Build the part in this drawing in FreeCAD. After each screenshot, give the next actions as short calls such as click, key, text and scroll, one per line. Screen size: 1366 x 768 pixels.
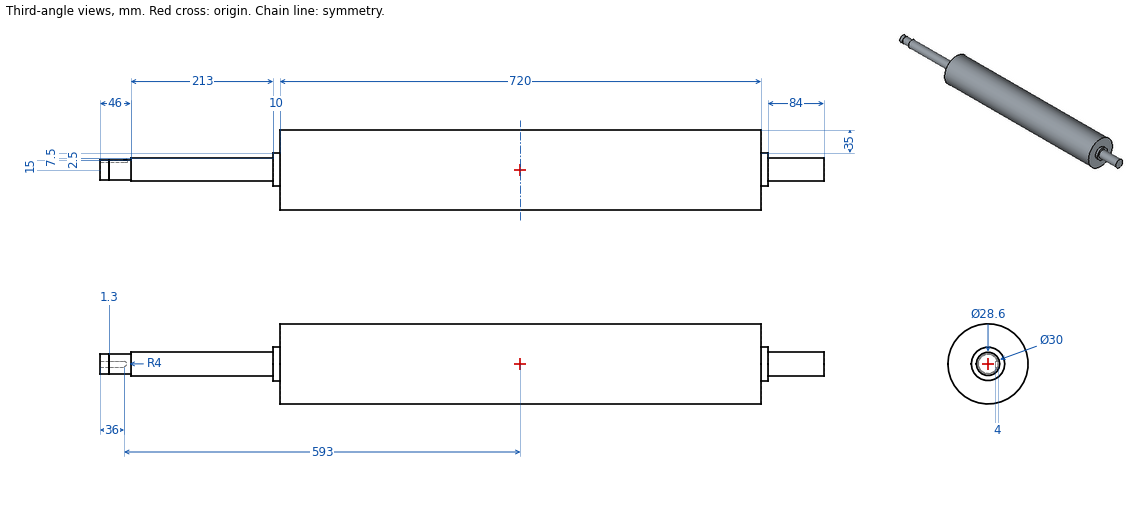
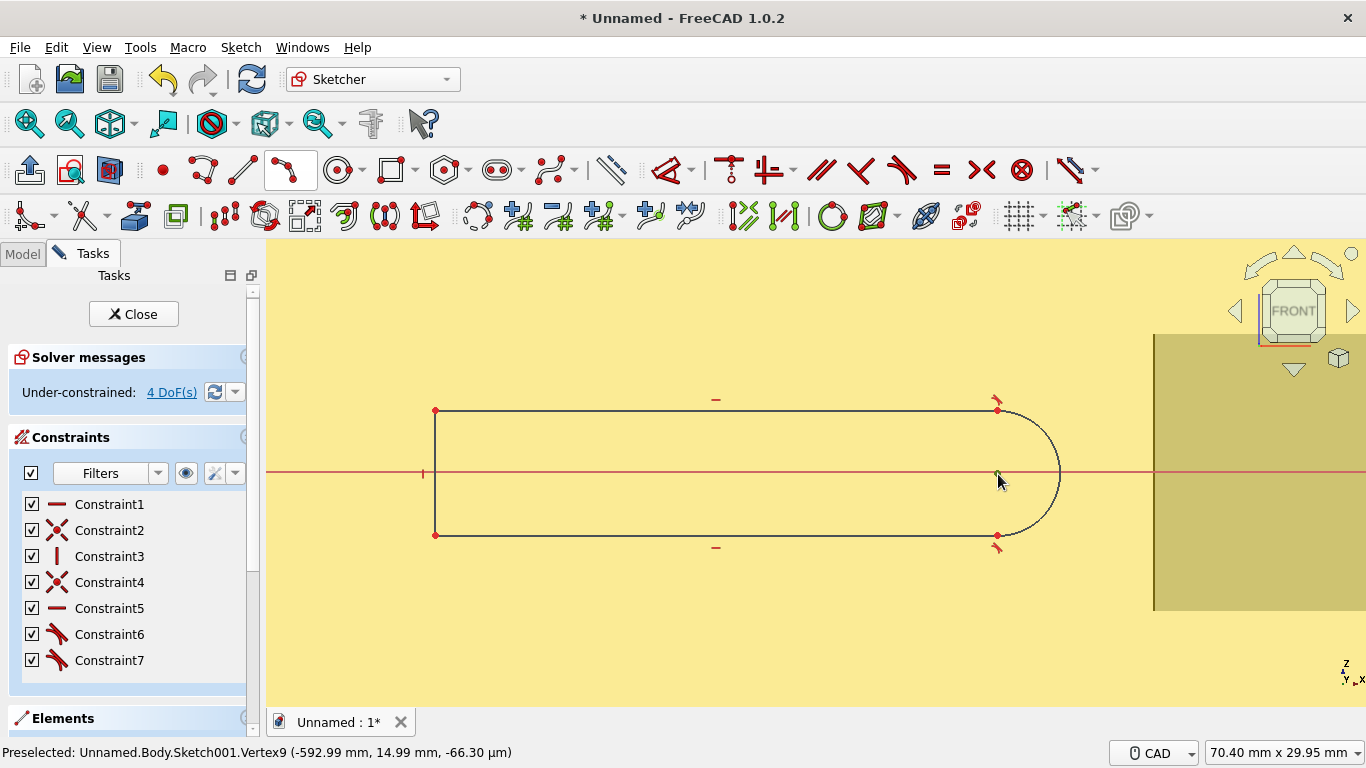
click(359, 472)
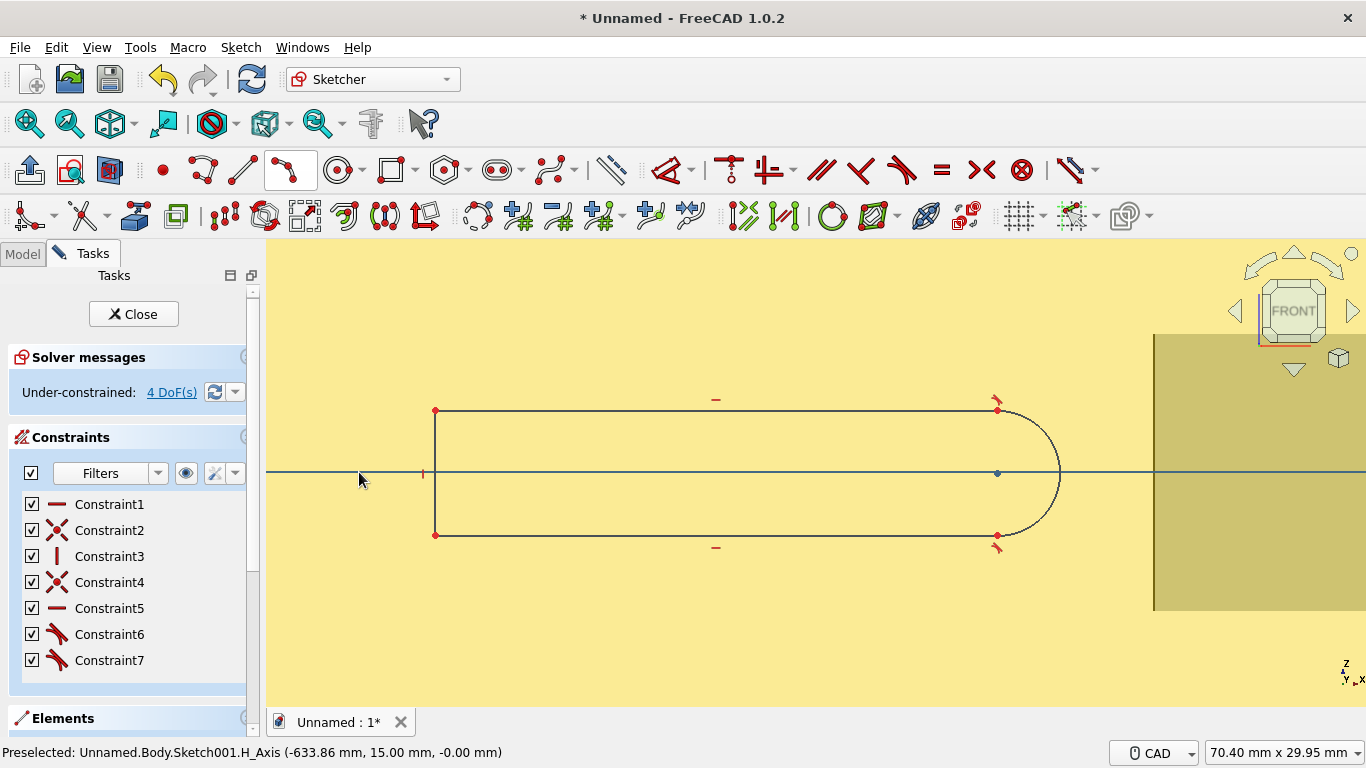
click(730, 170)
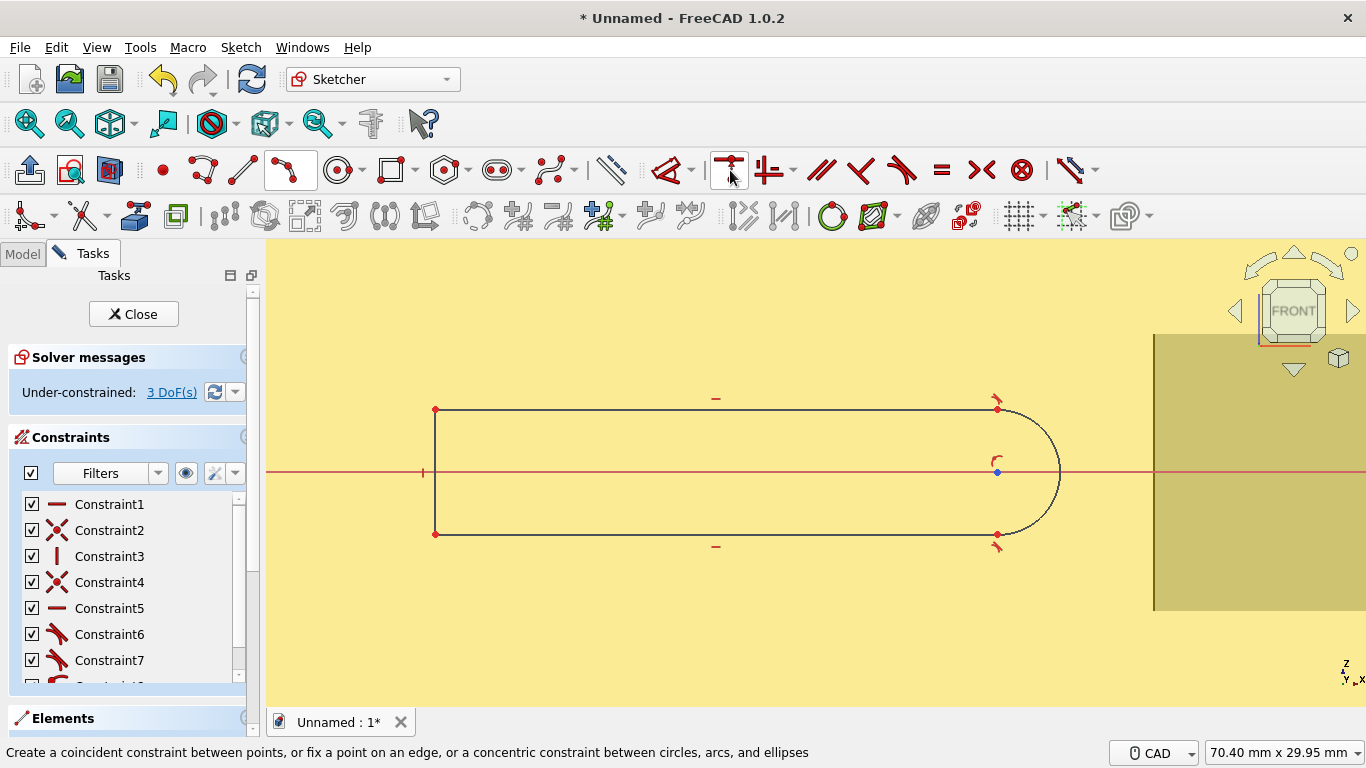
click(666, 170)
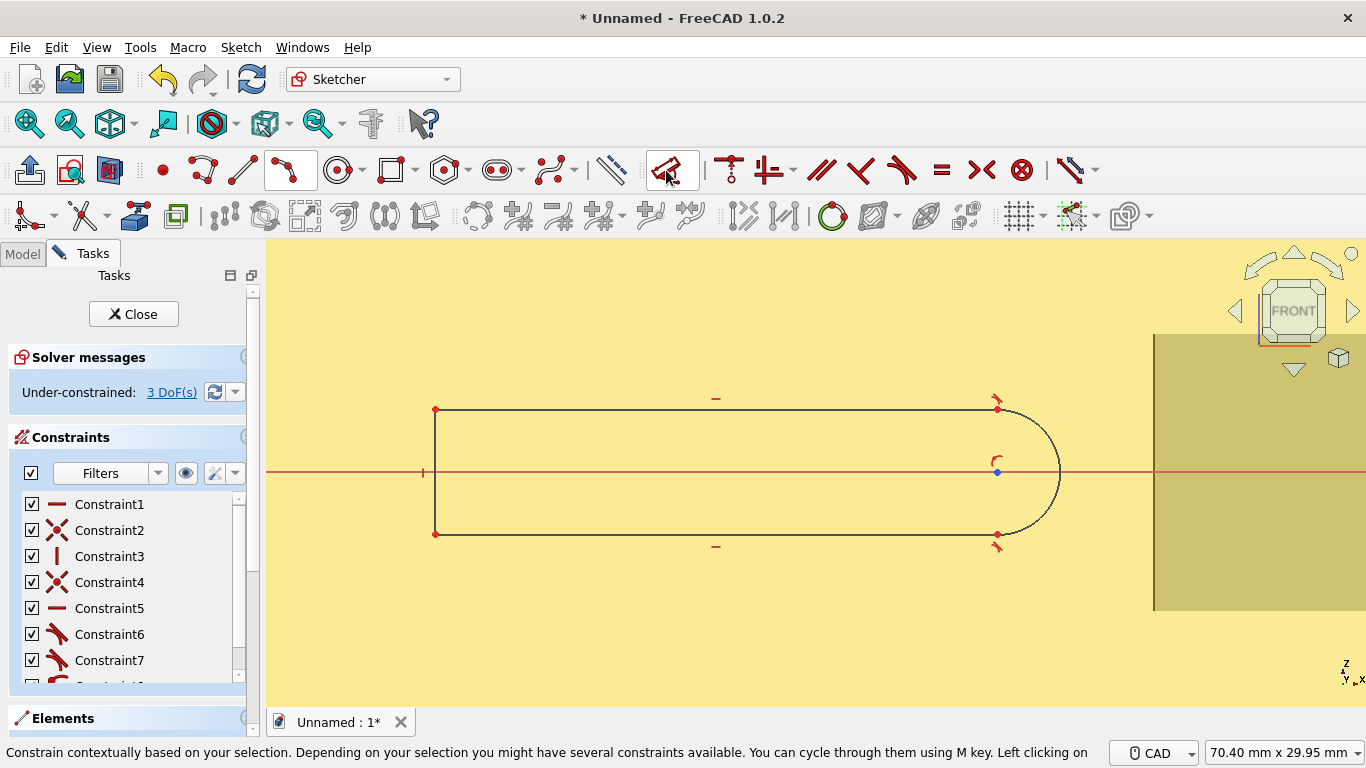
click(1048, 509)
click(1074, 528)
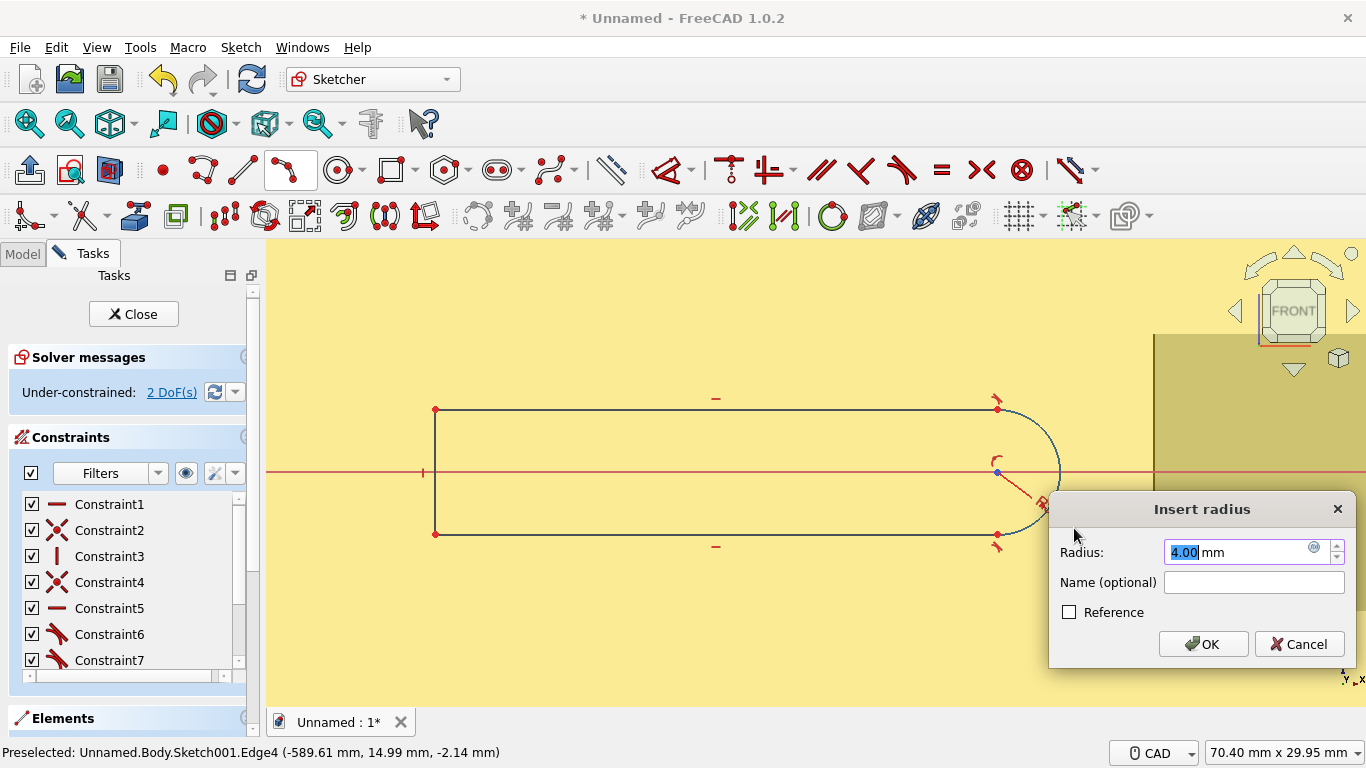
text(4)
key(Return)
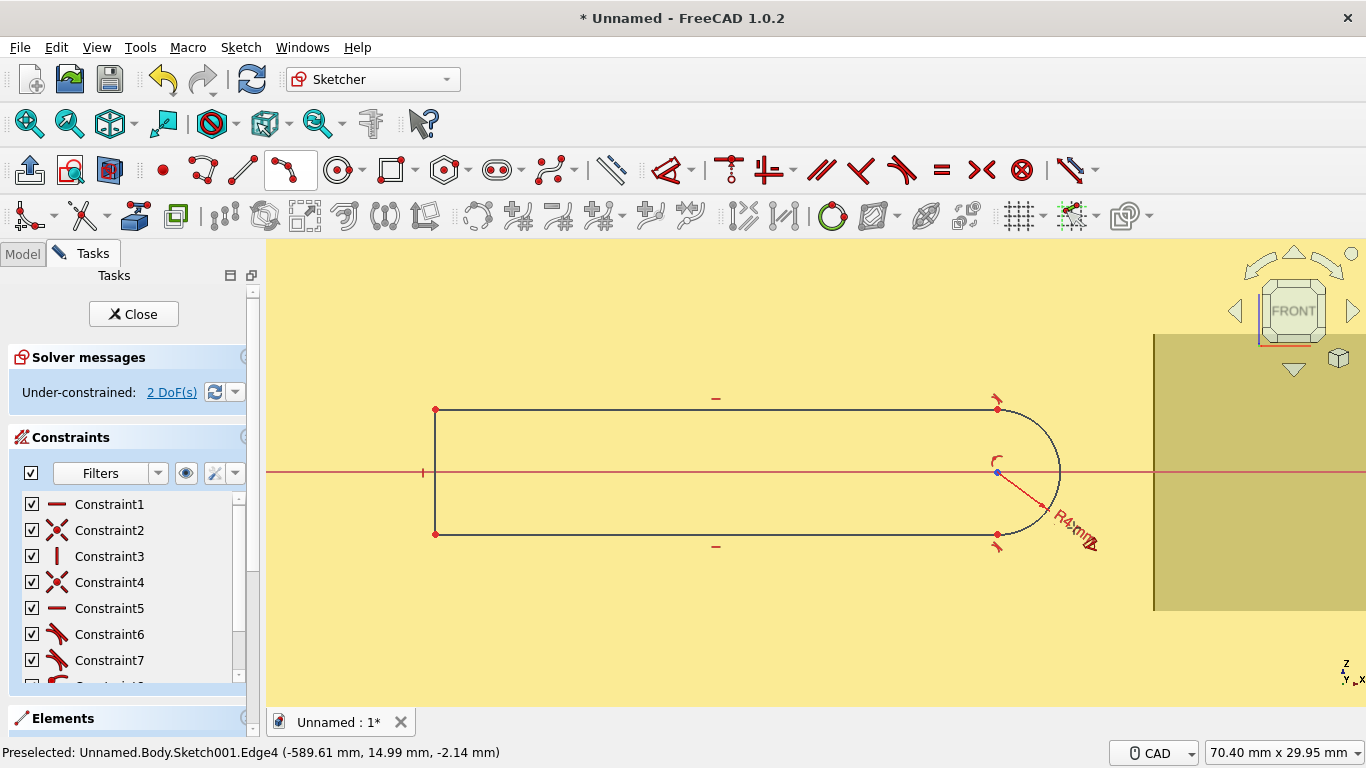
click(829, 535)
click(716, 569)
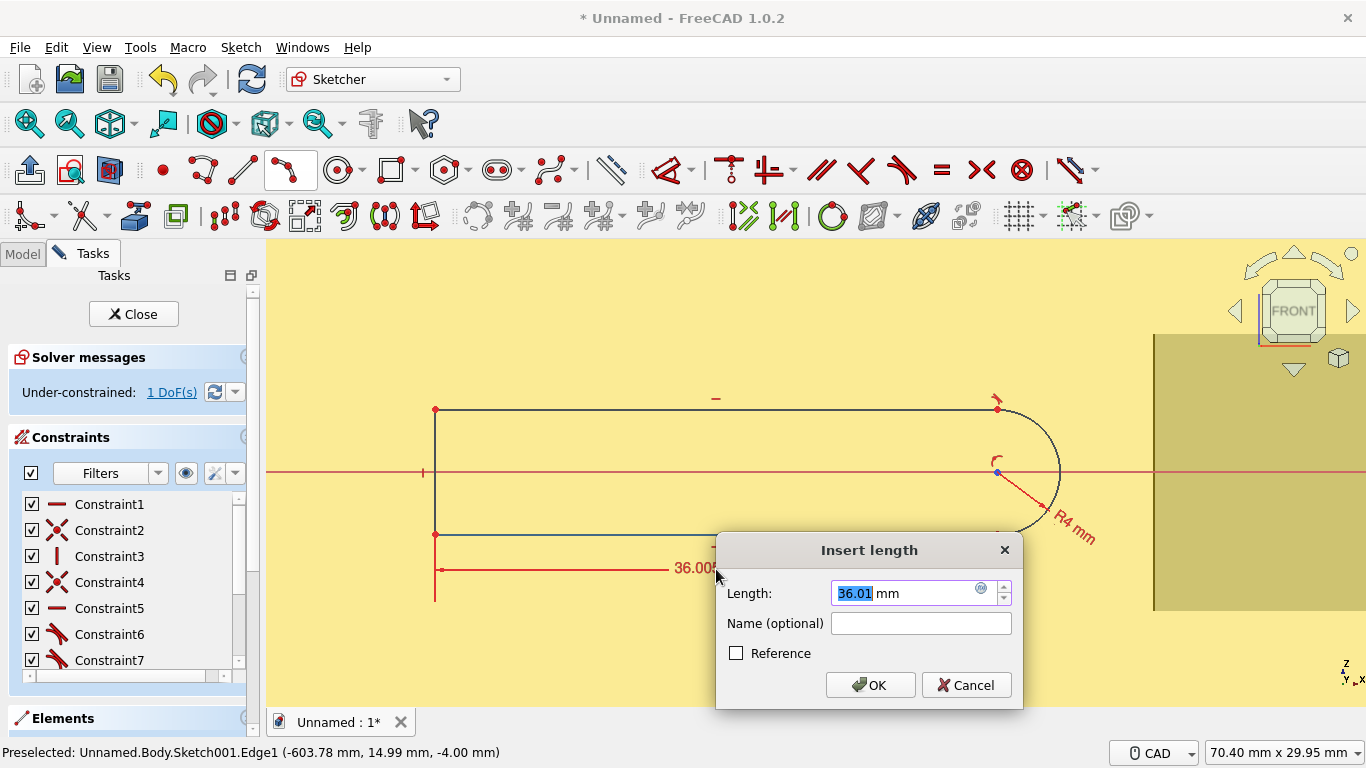
text(36)
key(Return)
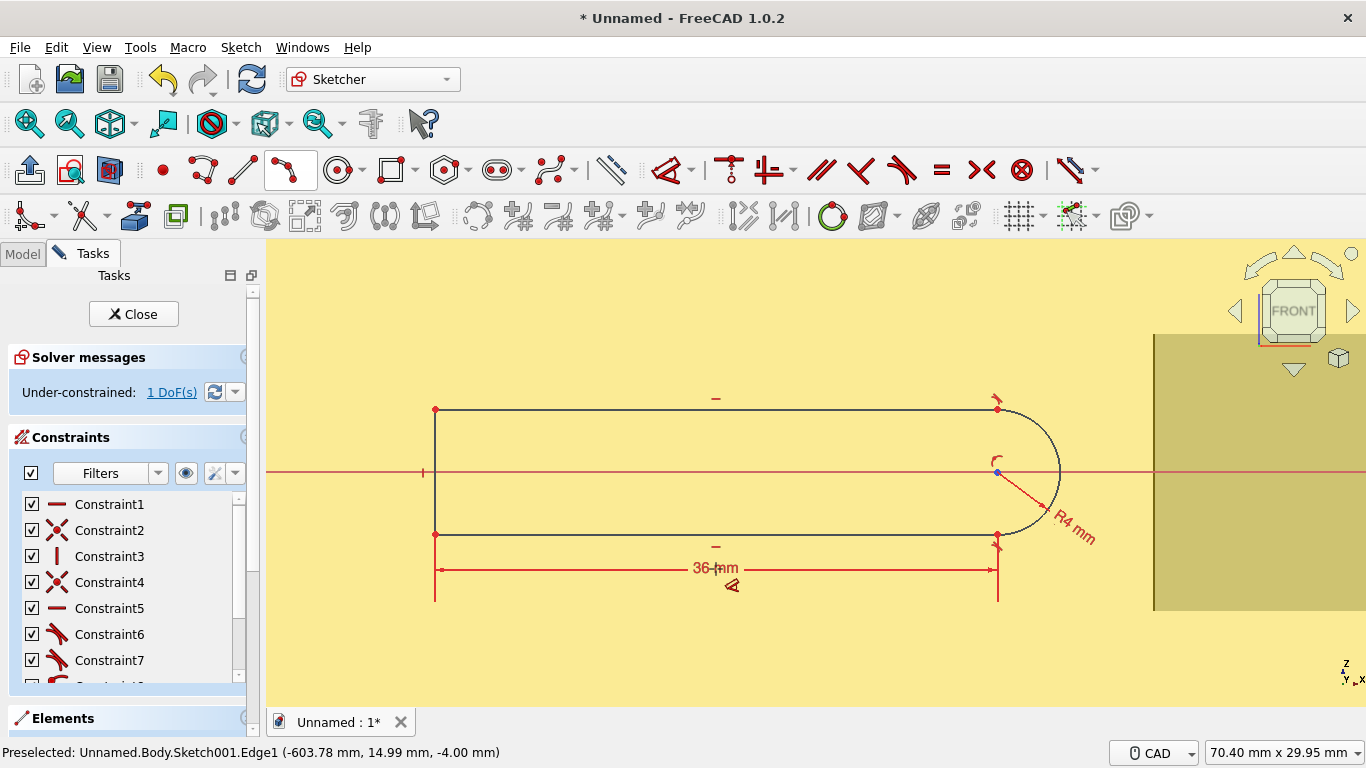
click(998, 535)
click(1099, 569)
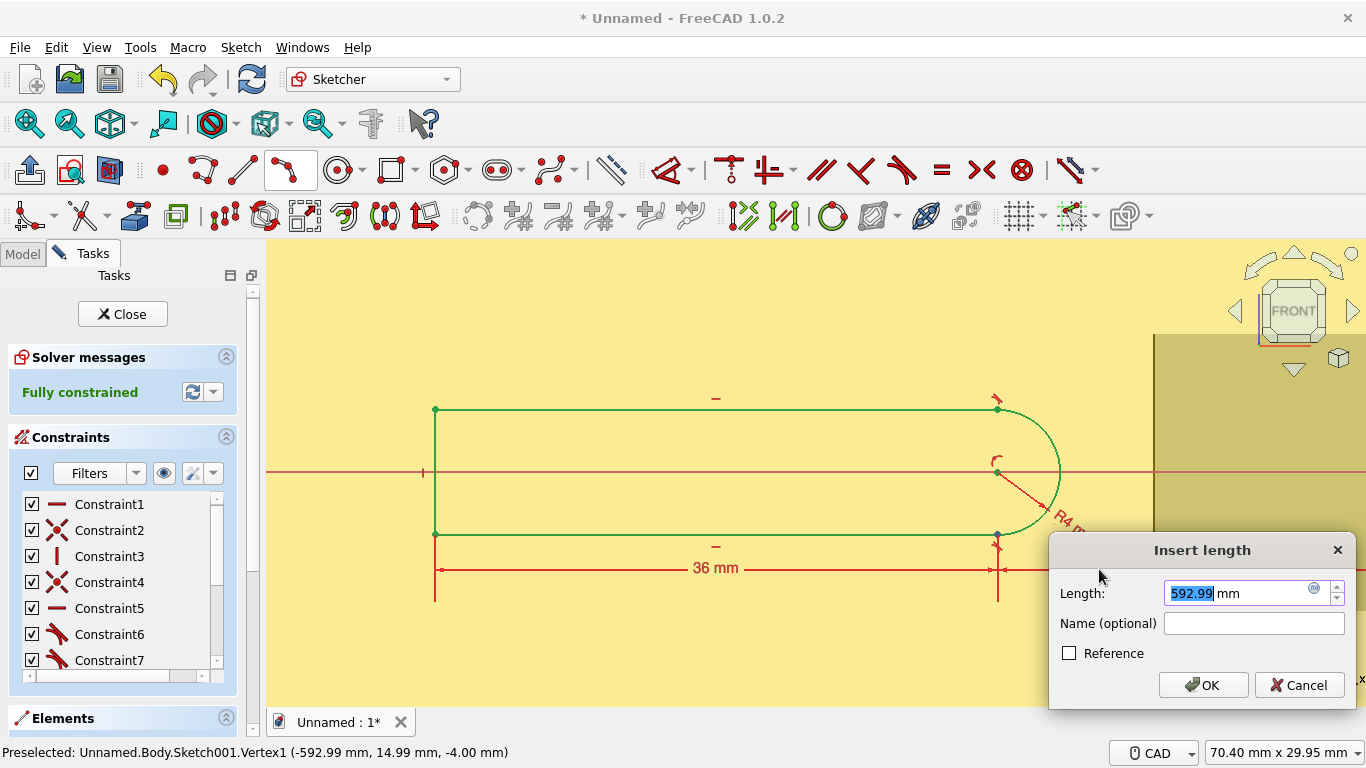
text(593)
key(Return)
key(Escape)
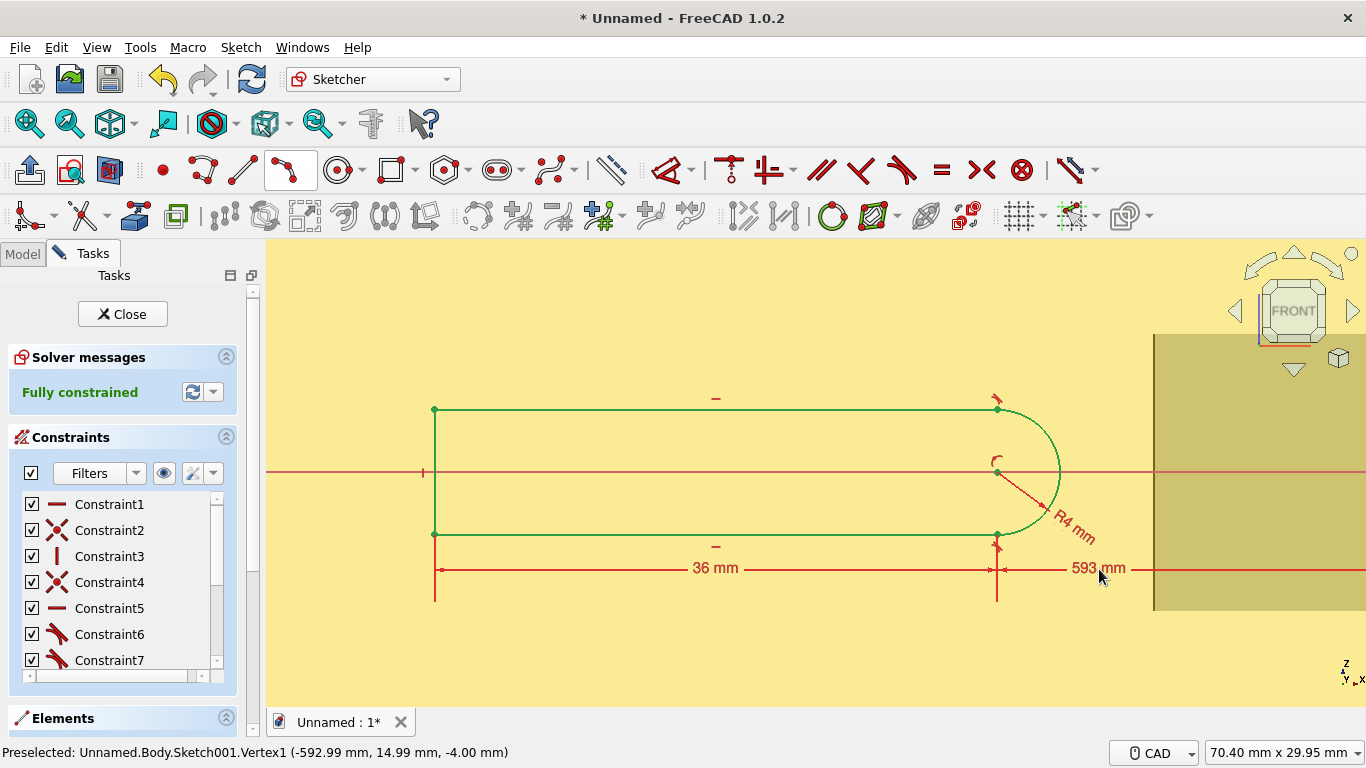
click(123, 314)